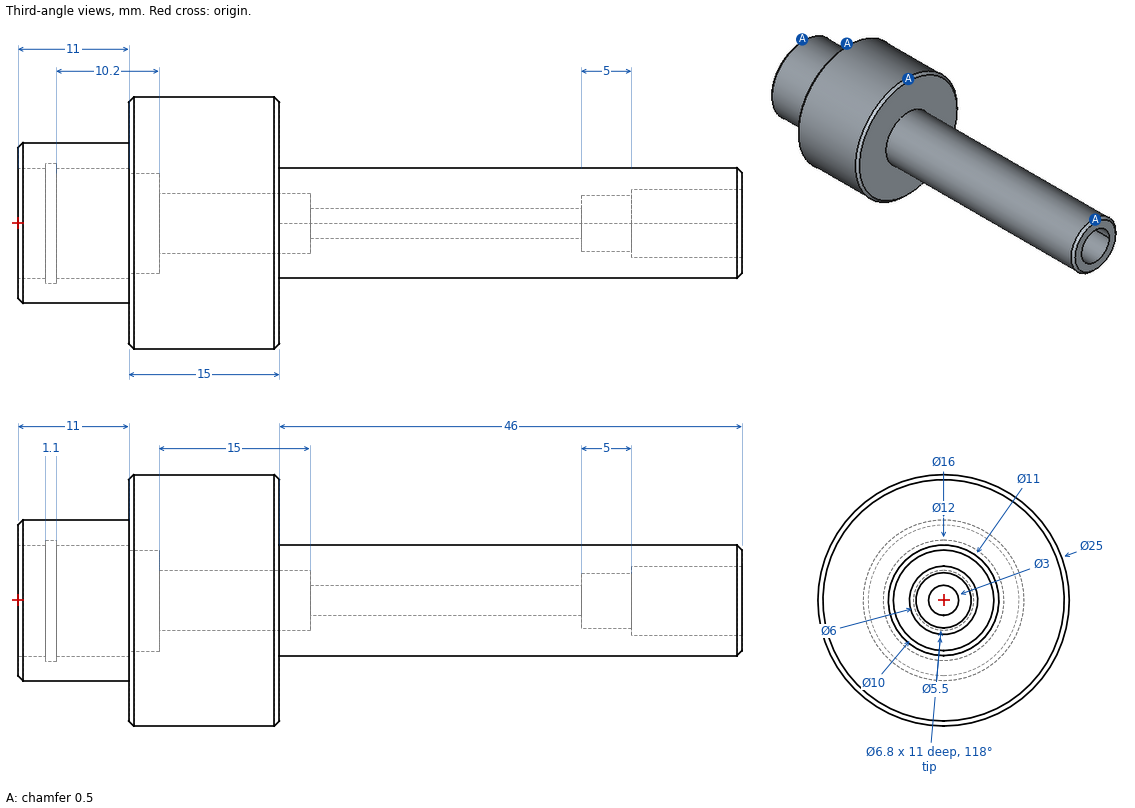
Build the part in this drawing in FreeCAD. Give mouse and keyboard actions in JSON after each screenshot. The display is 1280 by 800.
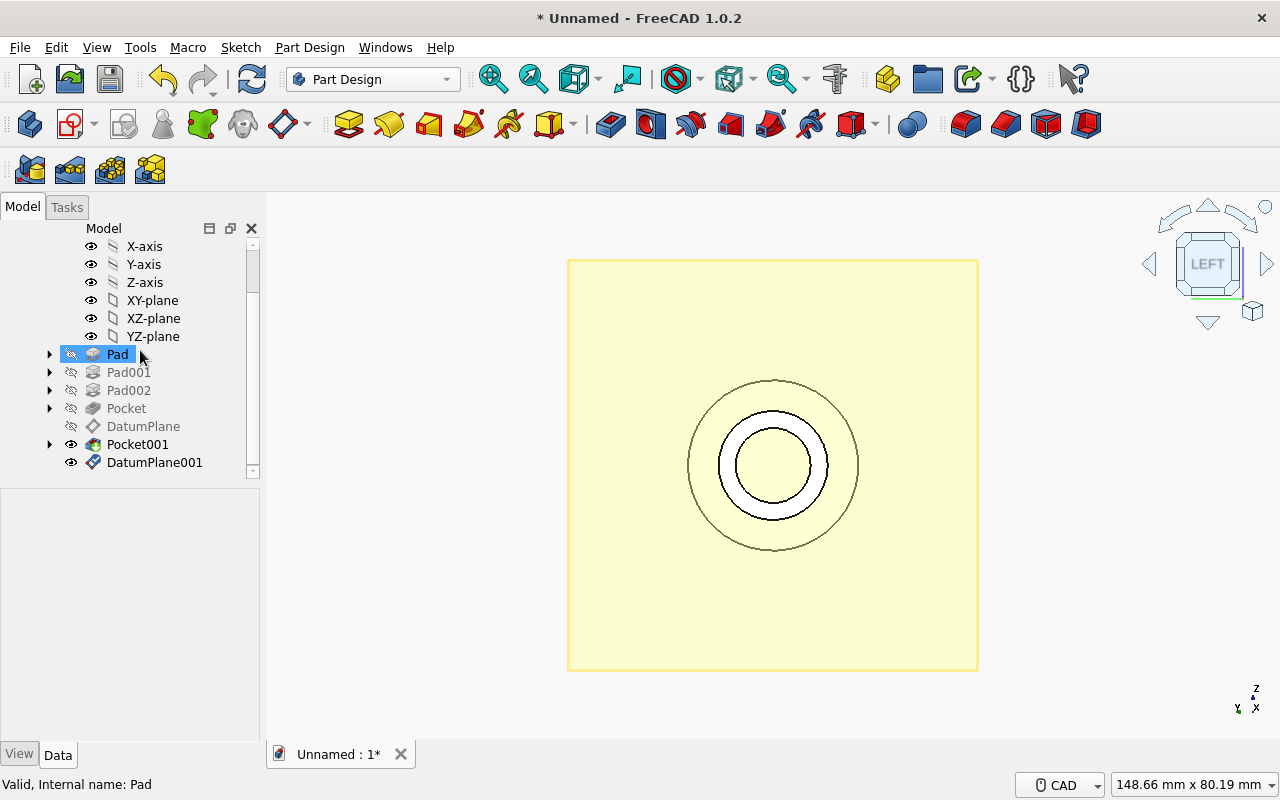
{"action": "left_click", "coordinate": [116, 462]}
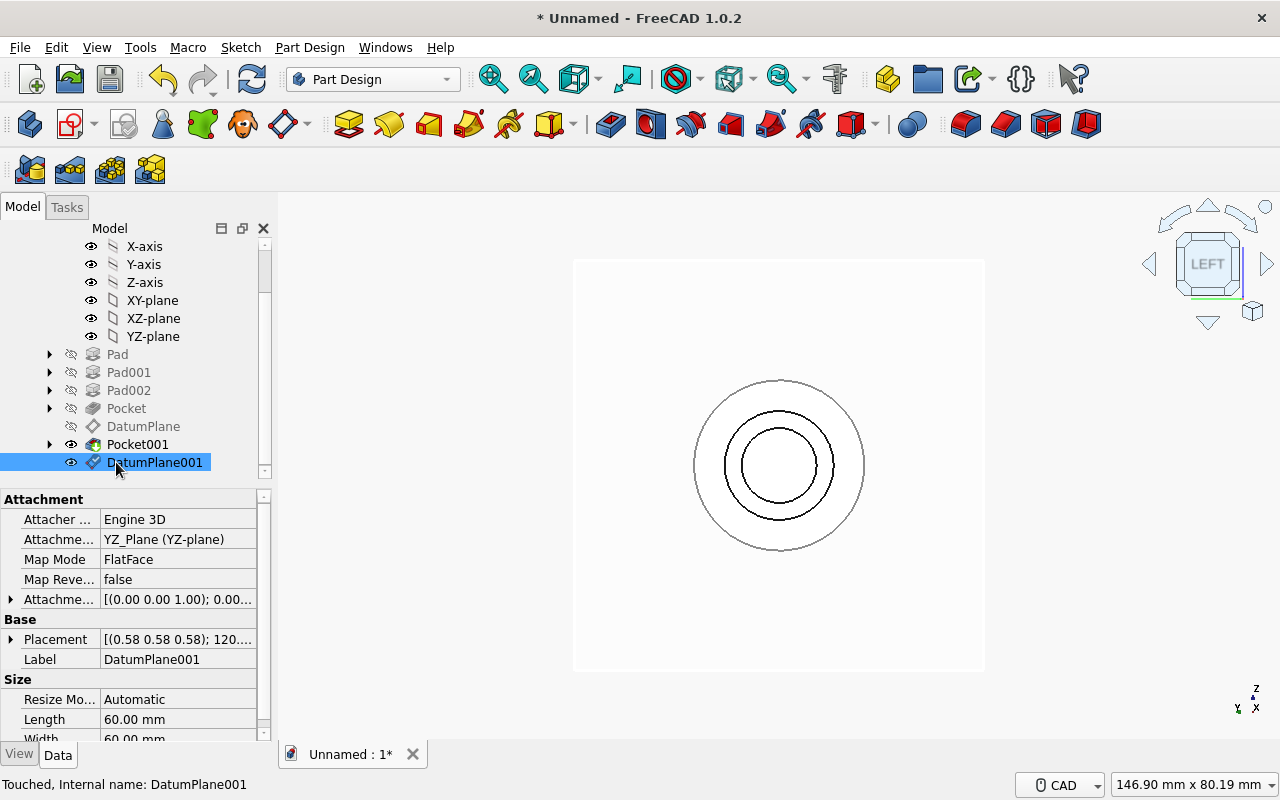
{"action": "left_click", "coordinate": [70, 124]}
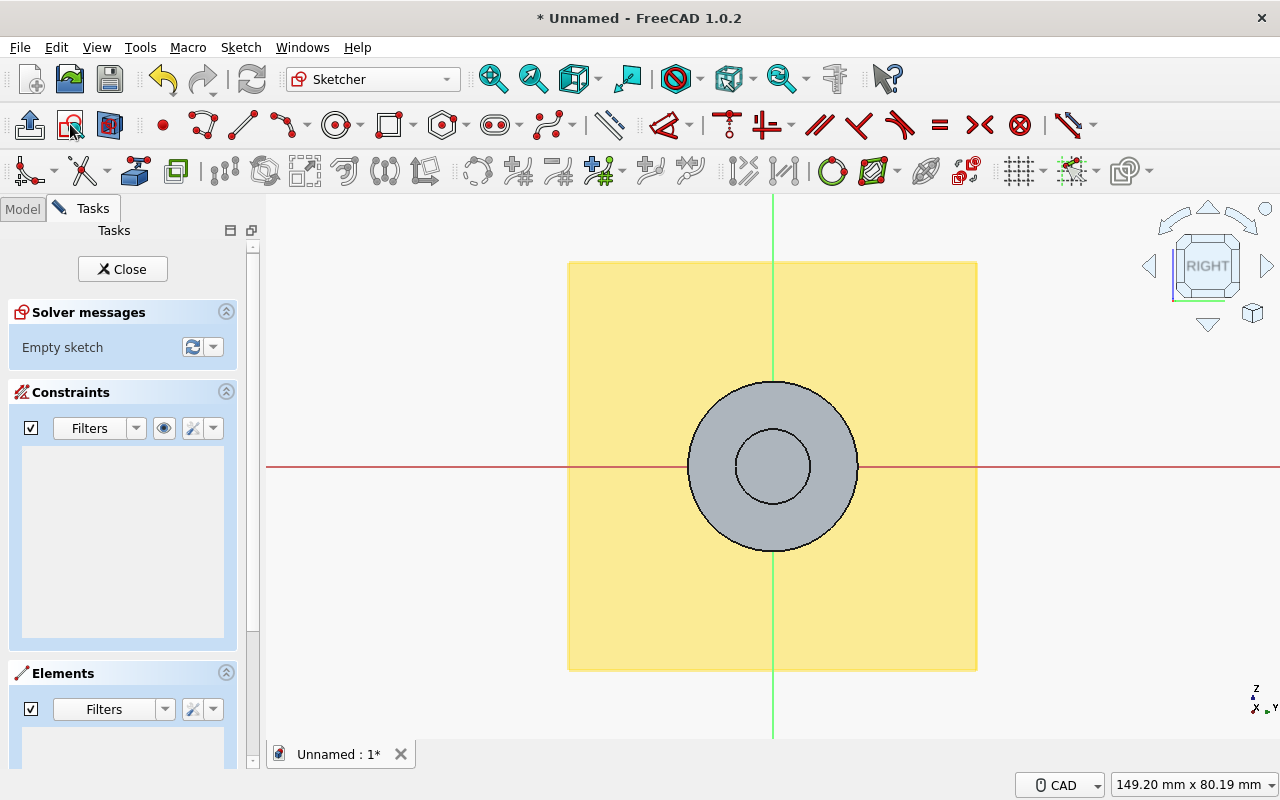
{"action": "key", "text": "q s"}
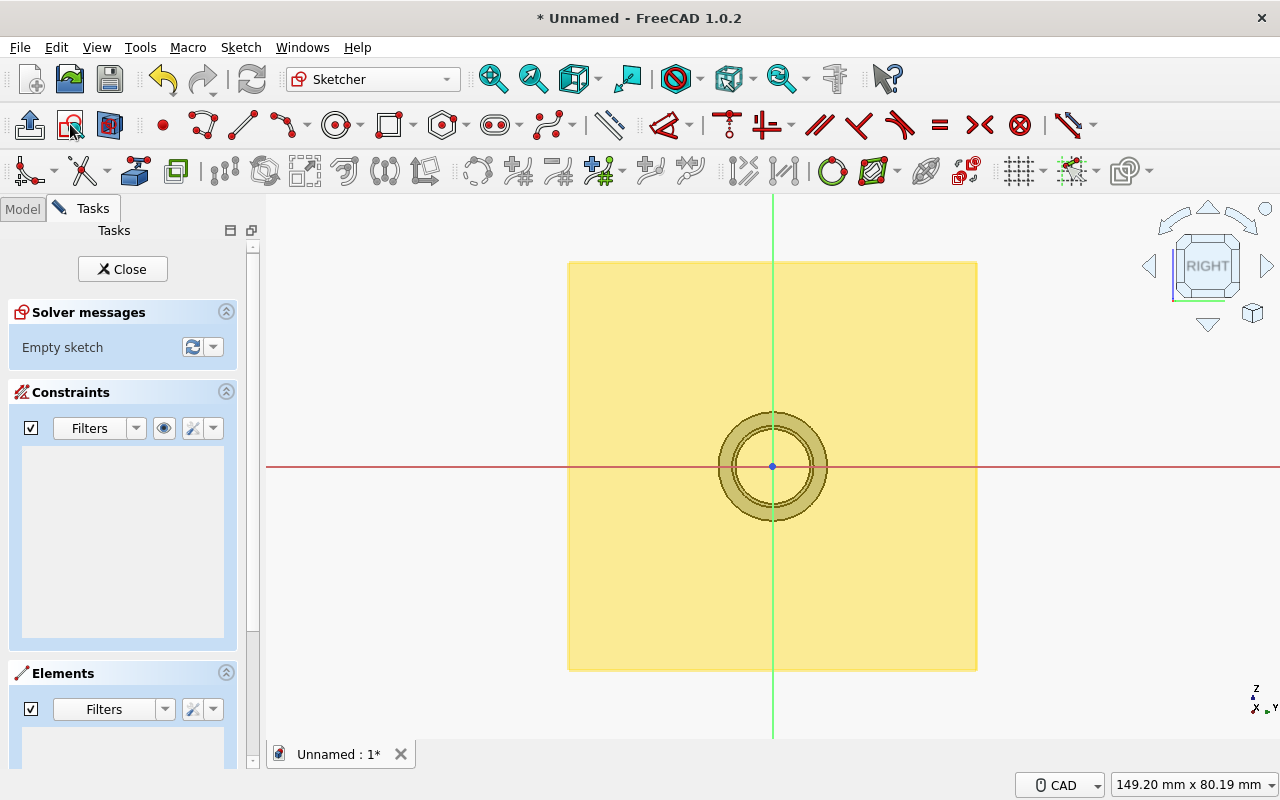
{"action": "scroll", "coordinate": [790, 466], "scroll_direction": "up", "scroll_amount": 8}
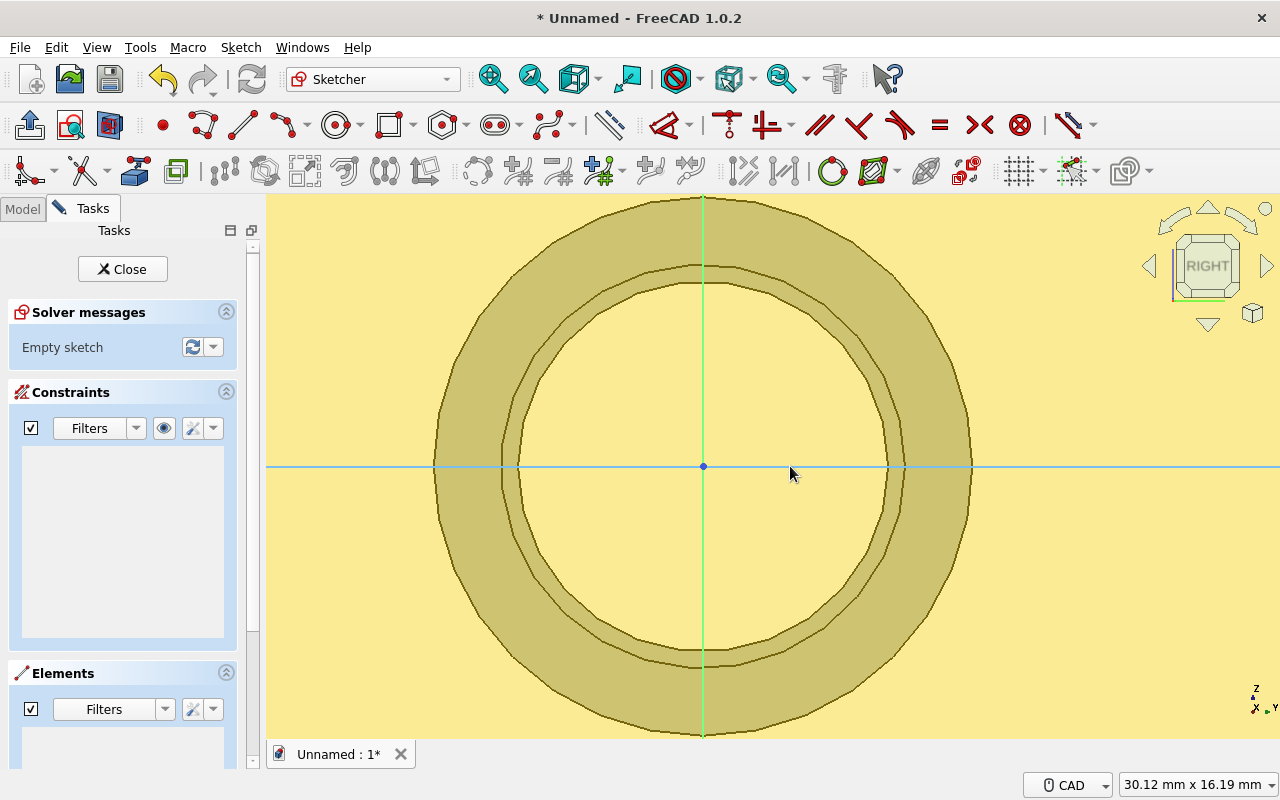
{"action": "left_click", "coordinate": [336, 126]}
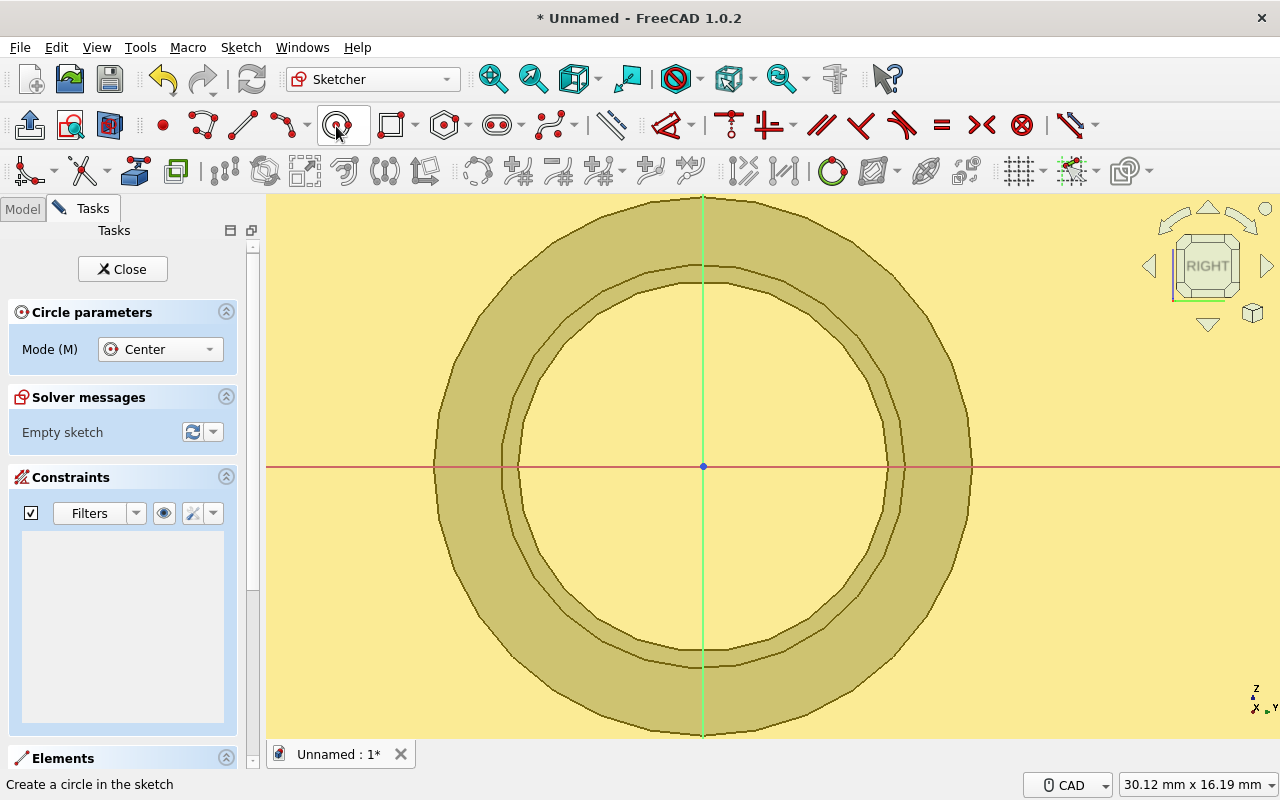
{"action": "left_click", "coordinate": [703, 466]}
{"action": "mouse_move", "coordinate": [822, 347]}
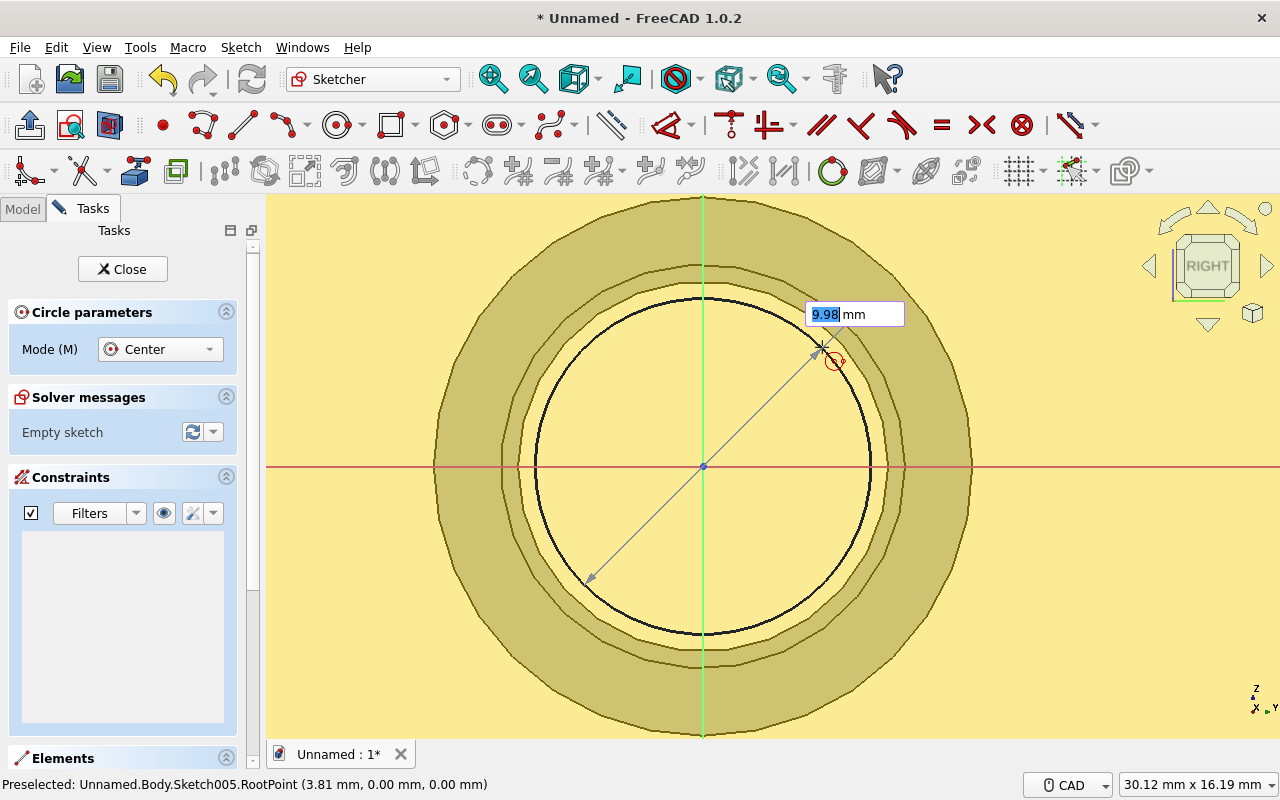
{"action": "type", "text": "10"}
{"action": "key", "text": "Return"}
{"action": "key", "text": "Escape"}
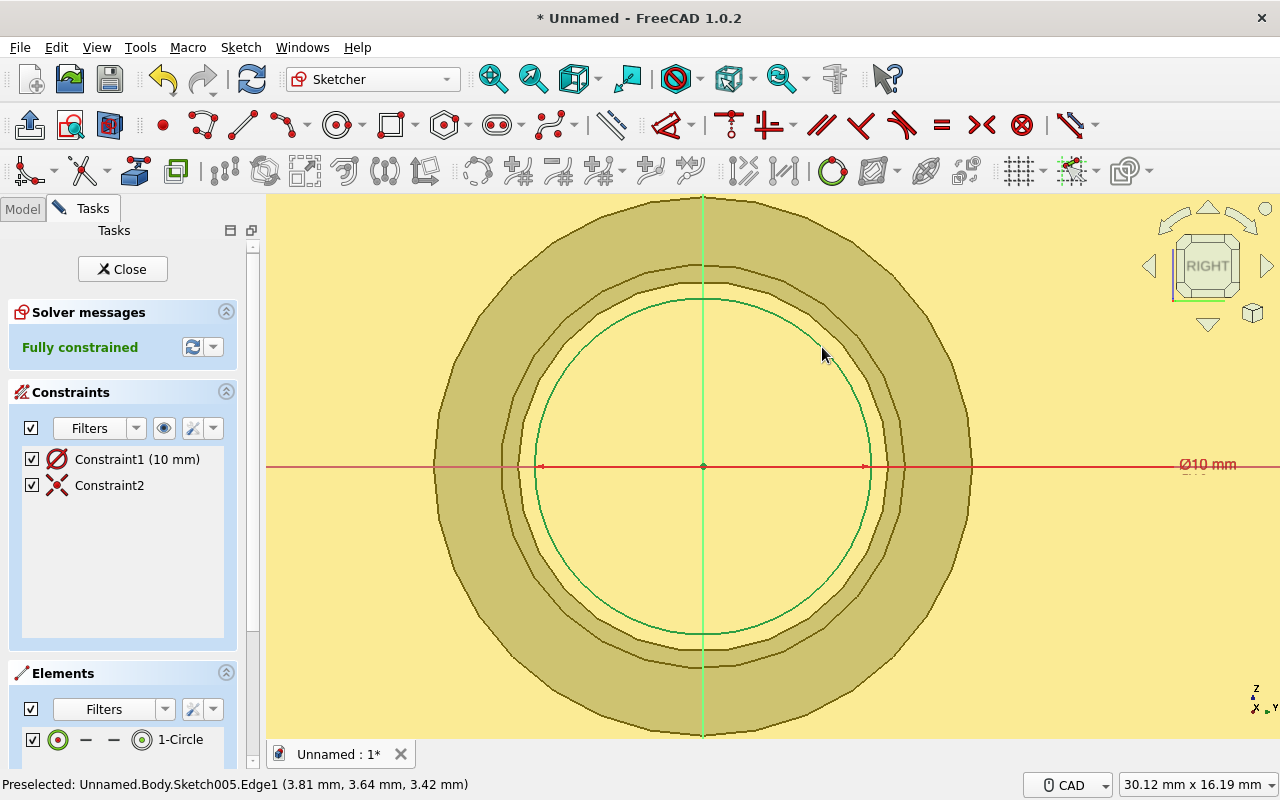
{"action": "left_click", "coordinate": [123, 269]}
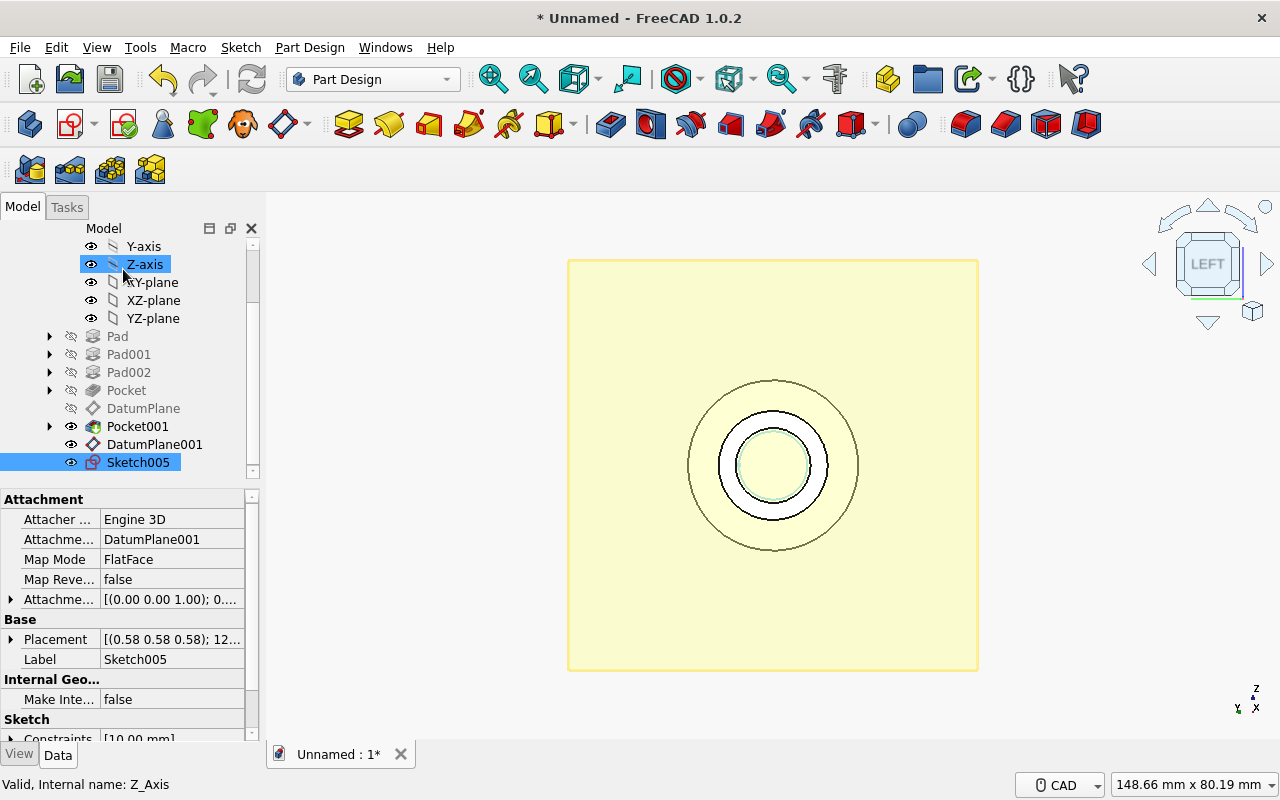
{"action": "left_click", "coordinate": [612, 124]}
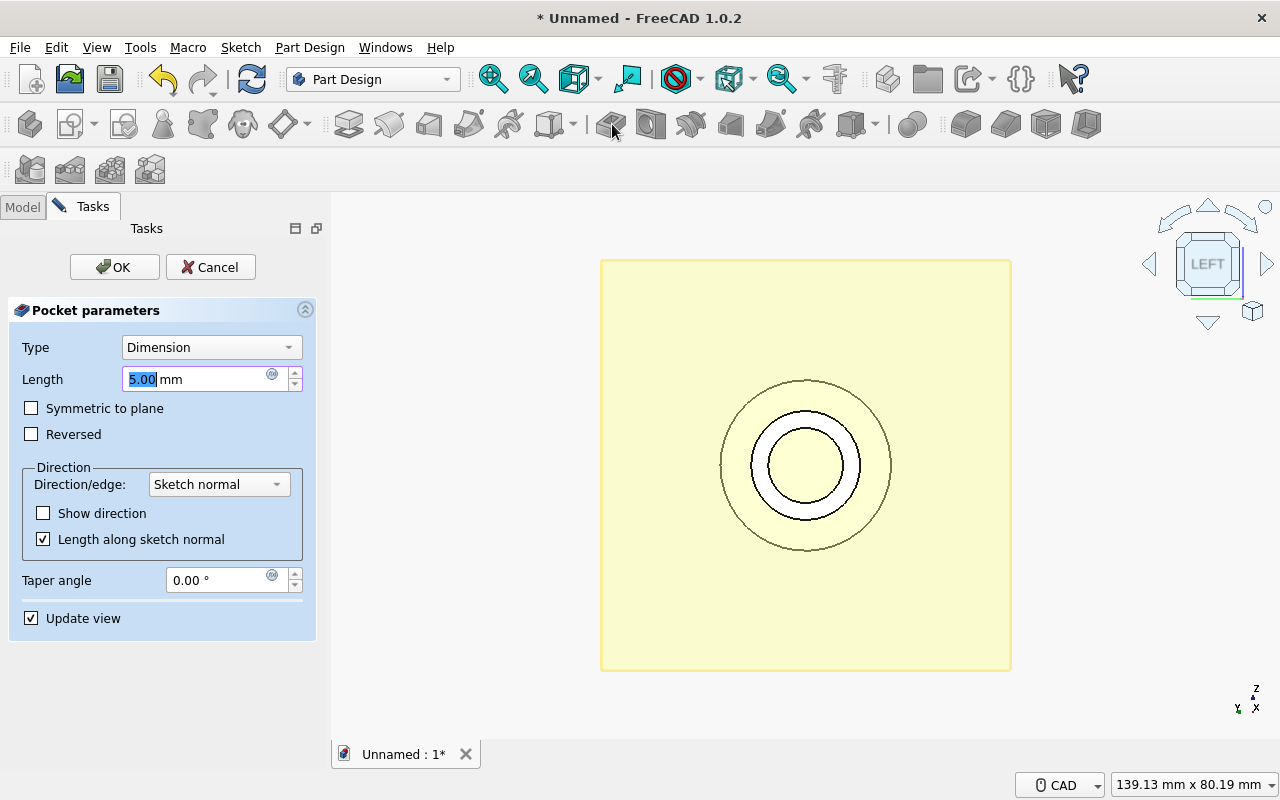
{"action": "type", "text": "10.2"}
{"action": "key", "text": "Tab"}